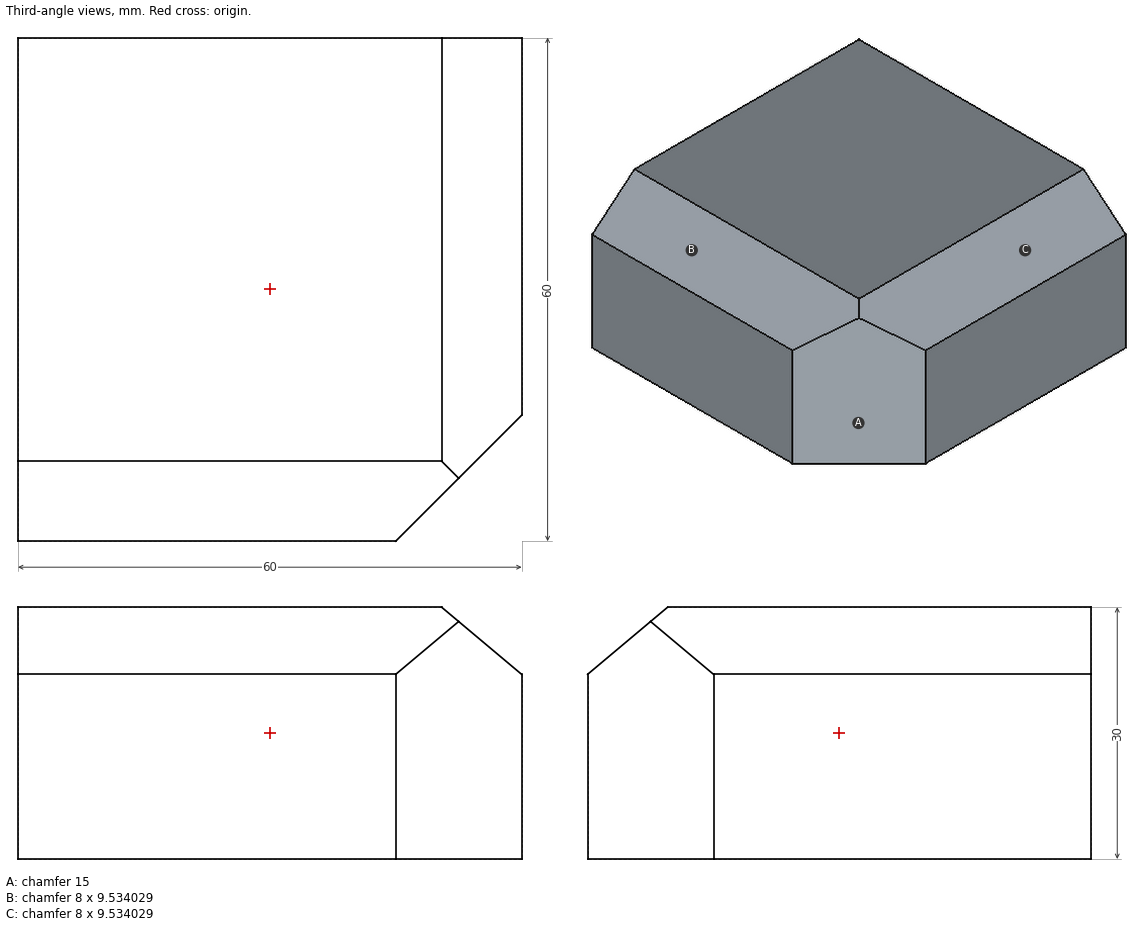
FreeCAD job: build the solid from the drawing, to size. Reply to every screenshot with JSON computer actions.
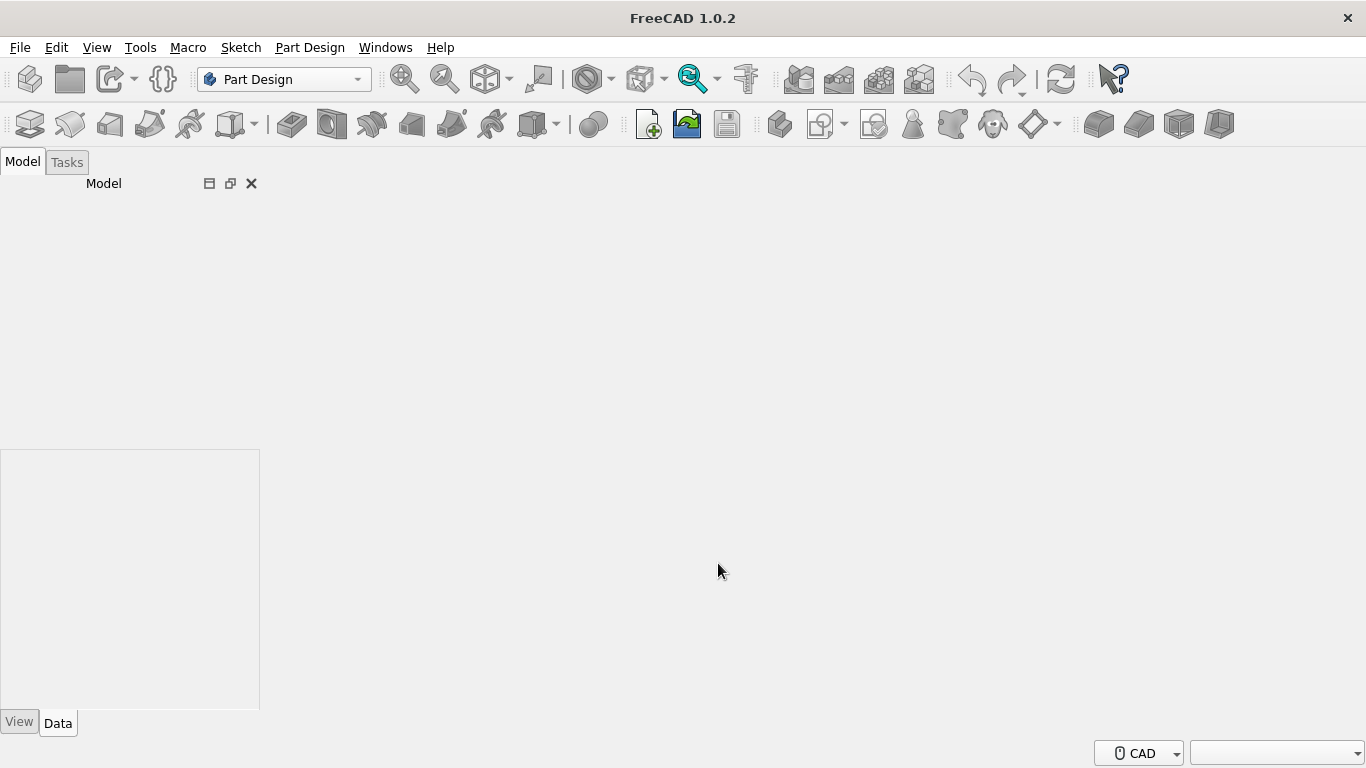
{"action": "key", "text": "ctrl+n"}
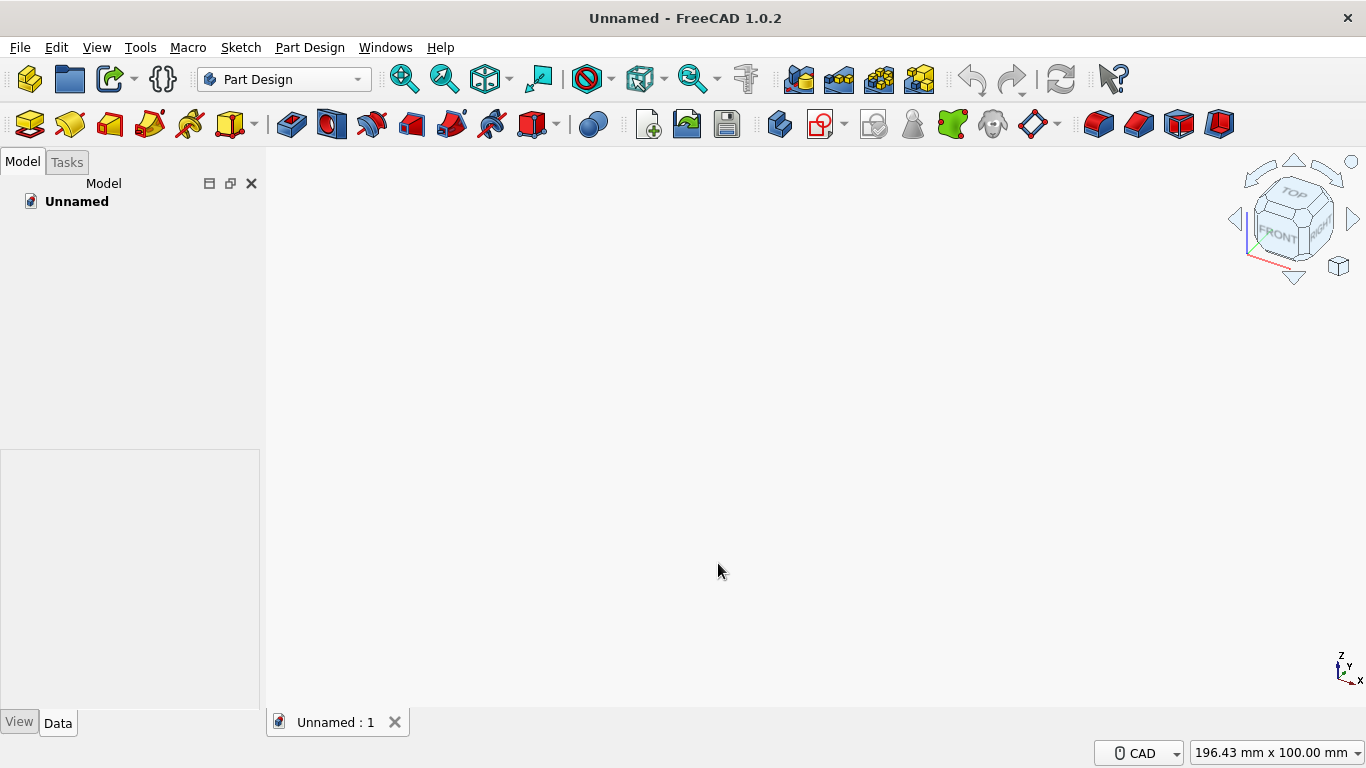
{"action": "left_click", "coordinate": [820, 124]}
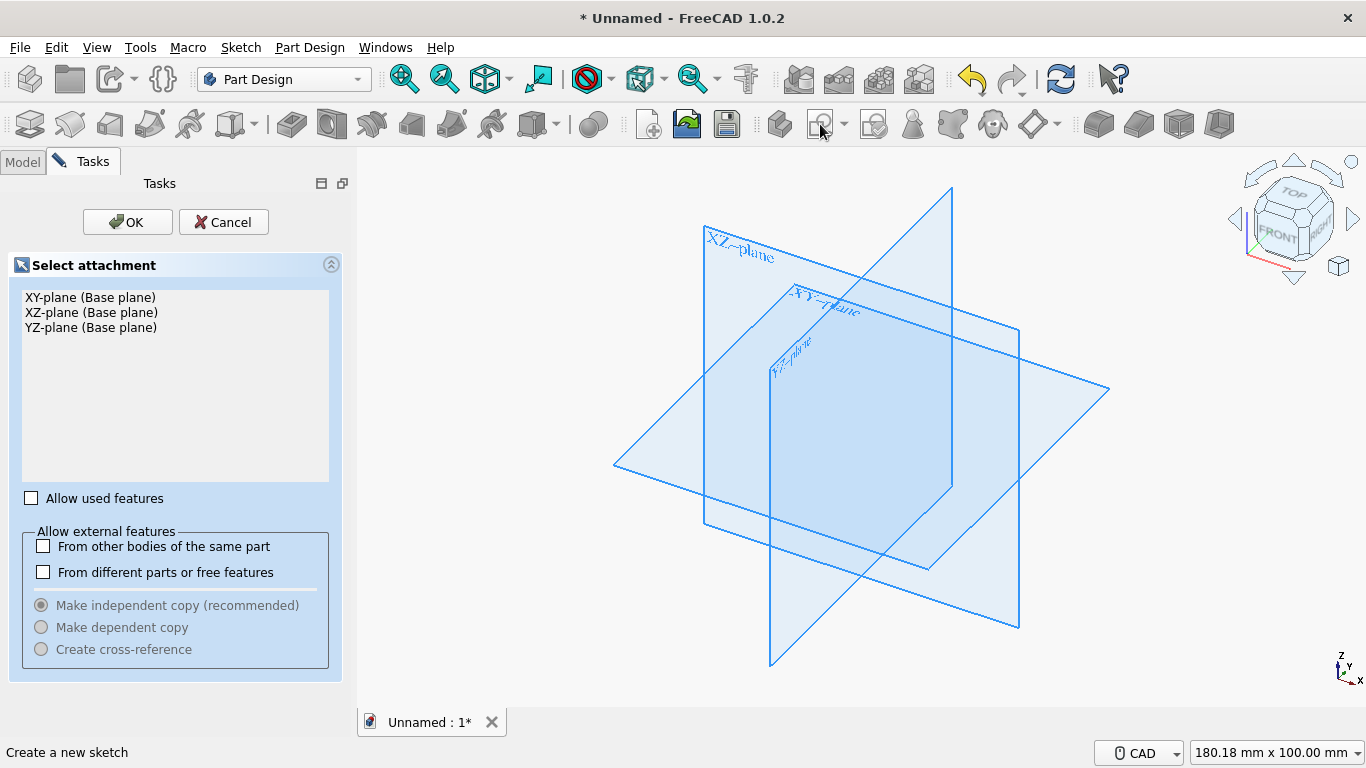
{"action": "left_click", "coordinate": [82, 298]}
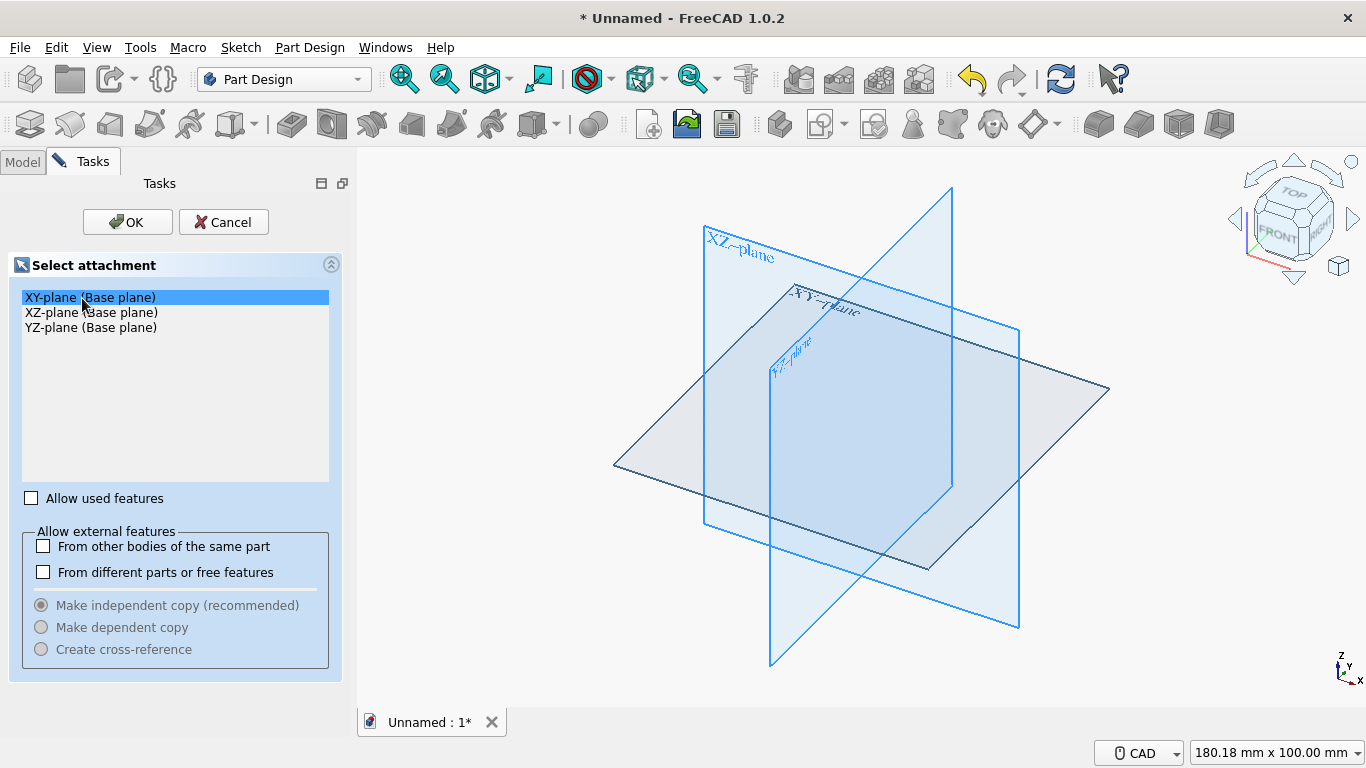
{"action": "left_click", "coordinate": [128, 222]}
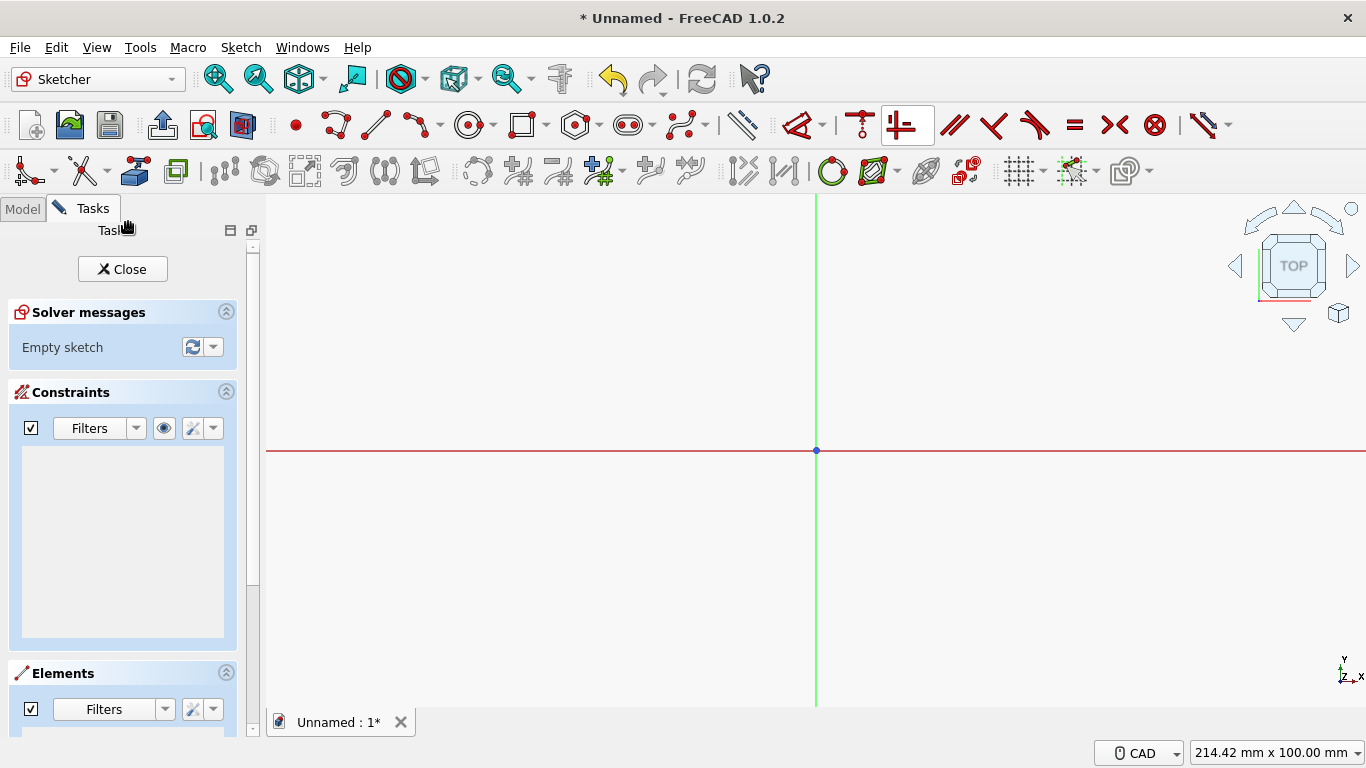
{"action": "key", "text": "g v"}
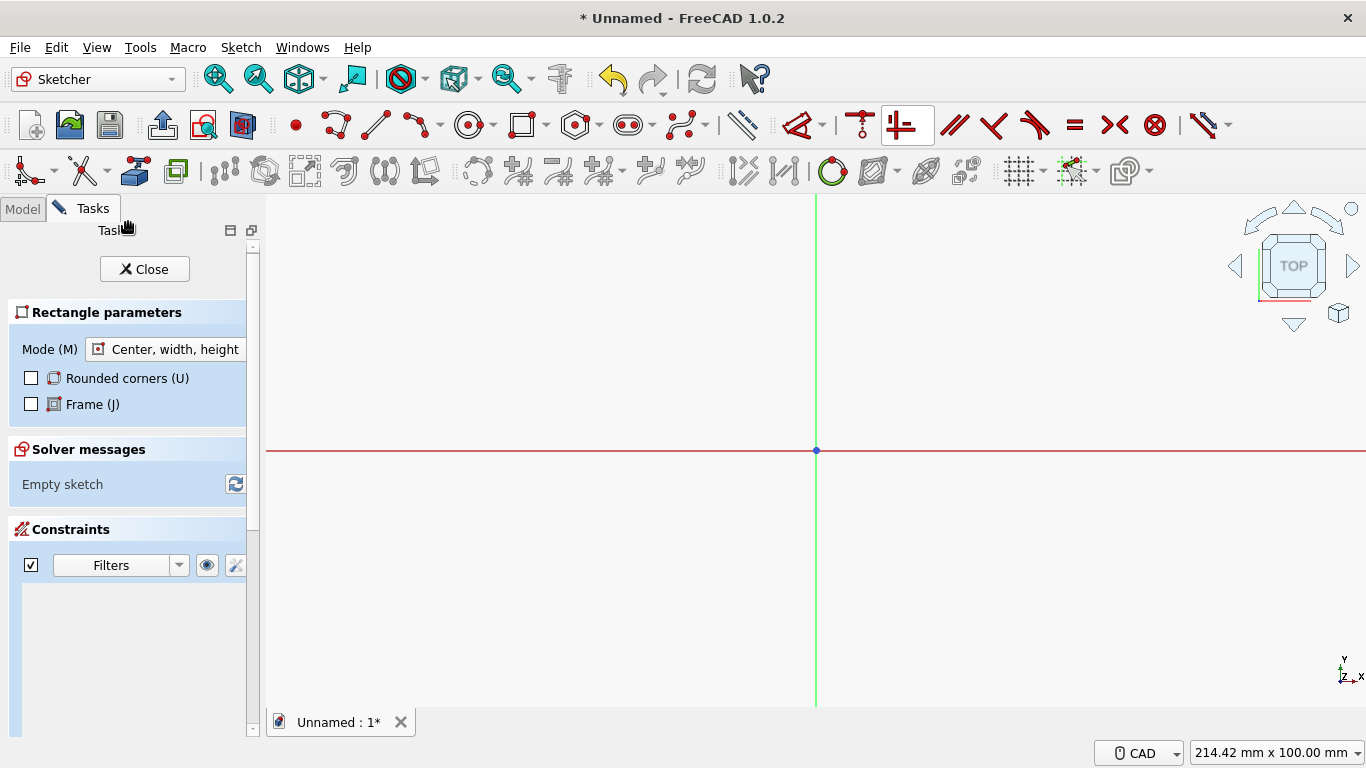
{"action": "left_click", "coordinate": [816, 450]}
{"action": "left_click", "coordinate": [970, 297]}
{"action": "key", "text": "Escape"}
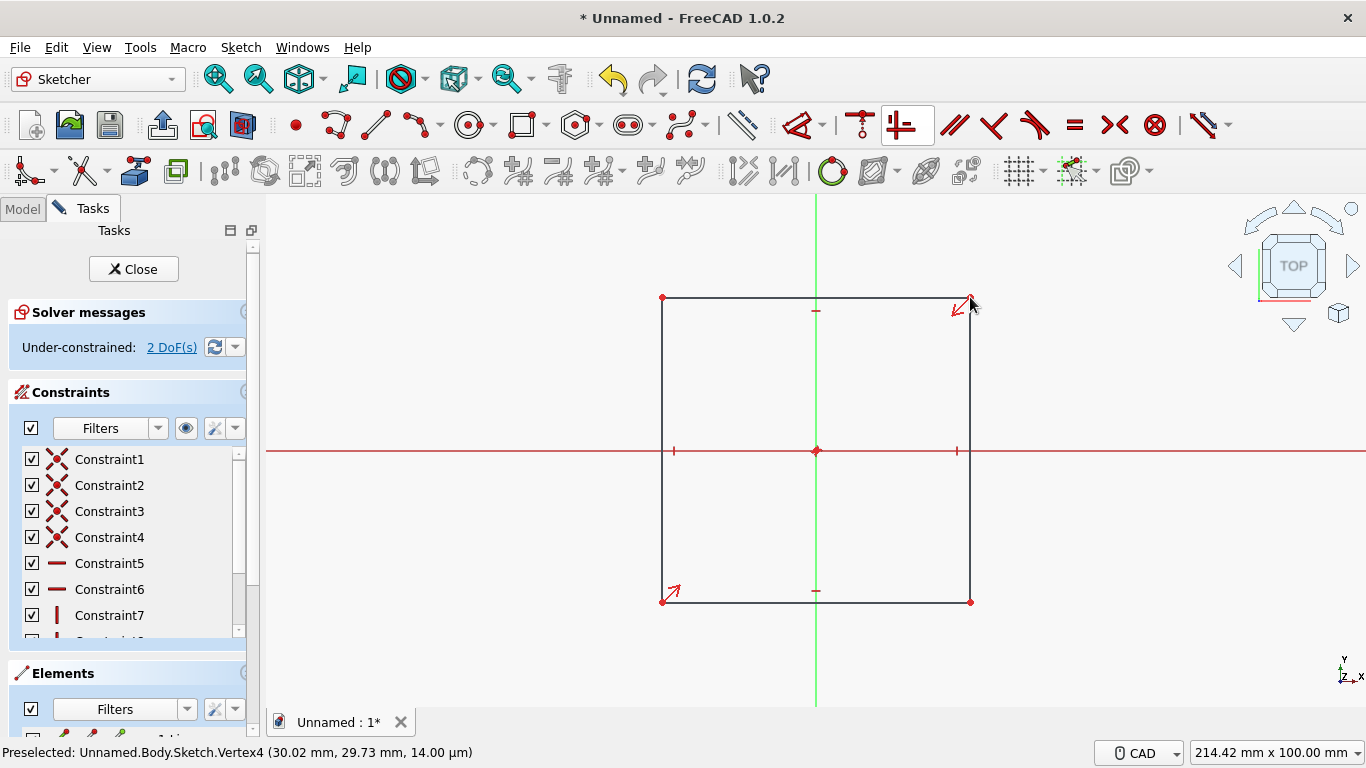
{"action": "left_click", "coordinate": [798, 126]}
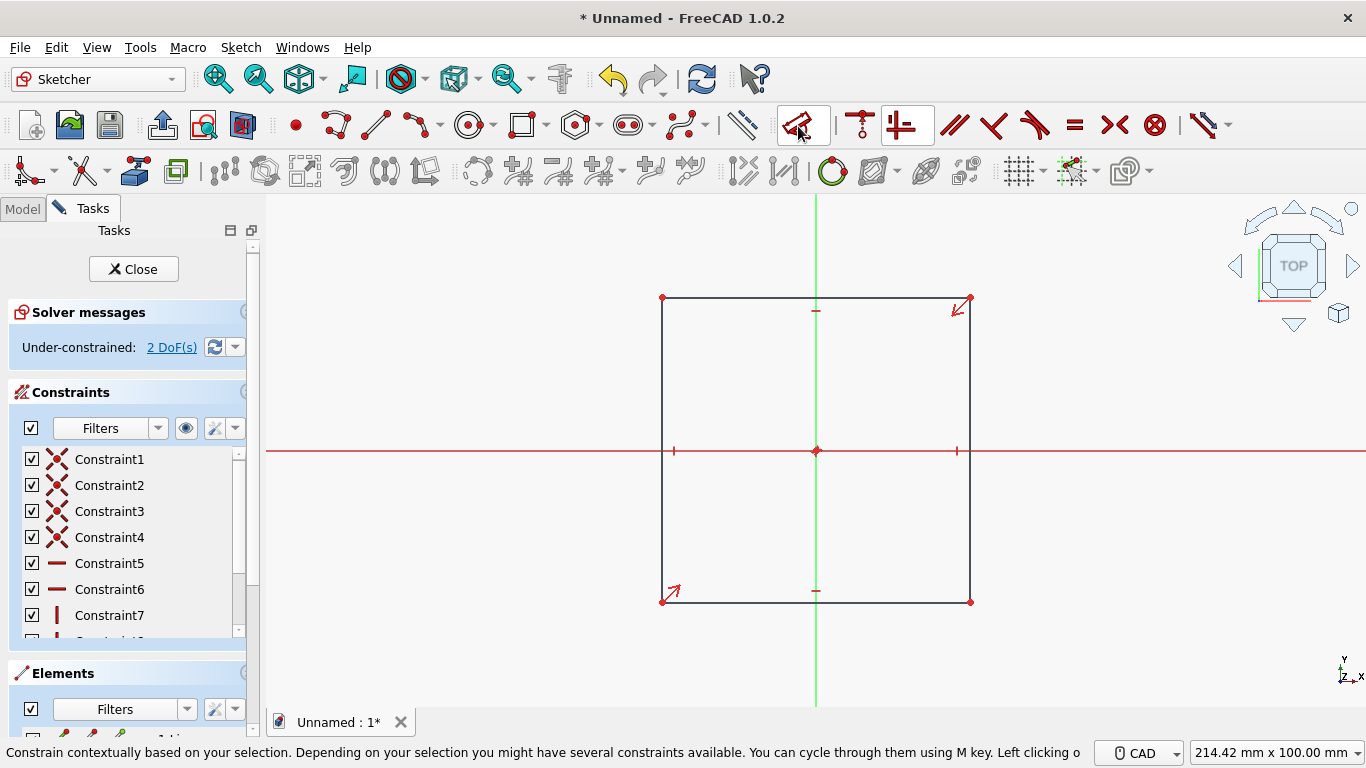
{"action": "left_click", "coordinate": [754, 603]}
{"action": "left_click", "coordinate": [745, 637]}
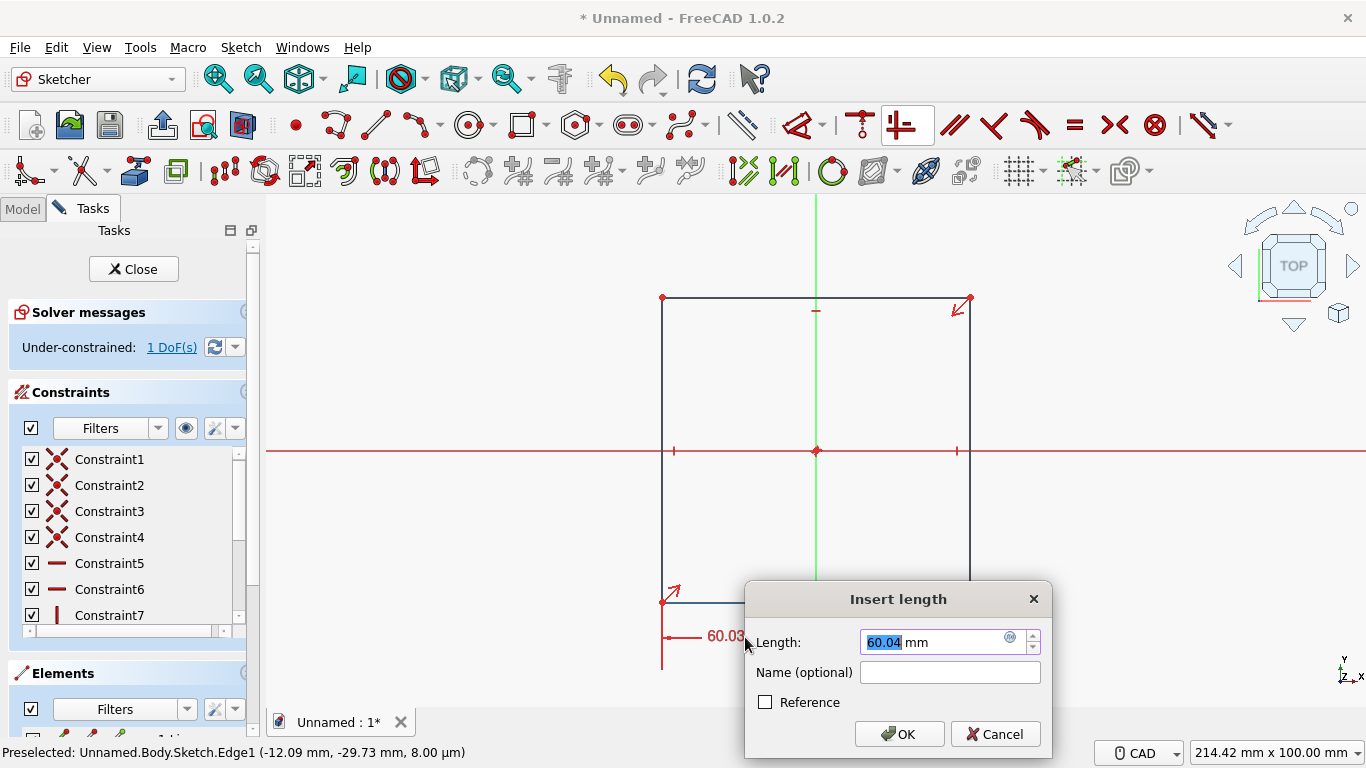
{"action": "type", "text": "60"}
{"action": "key", "text": "Return"}